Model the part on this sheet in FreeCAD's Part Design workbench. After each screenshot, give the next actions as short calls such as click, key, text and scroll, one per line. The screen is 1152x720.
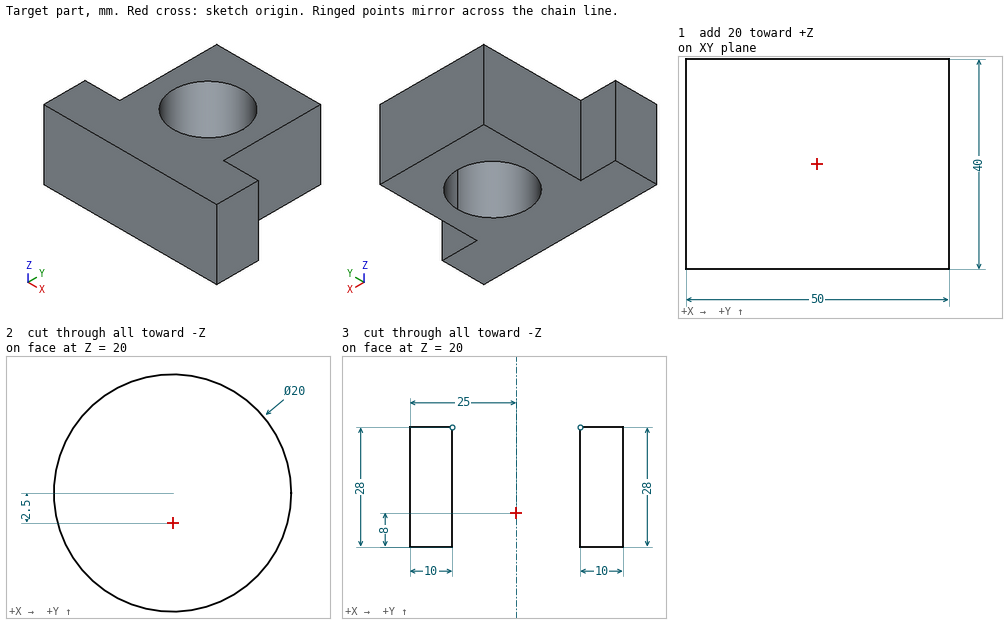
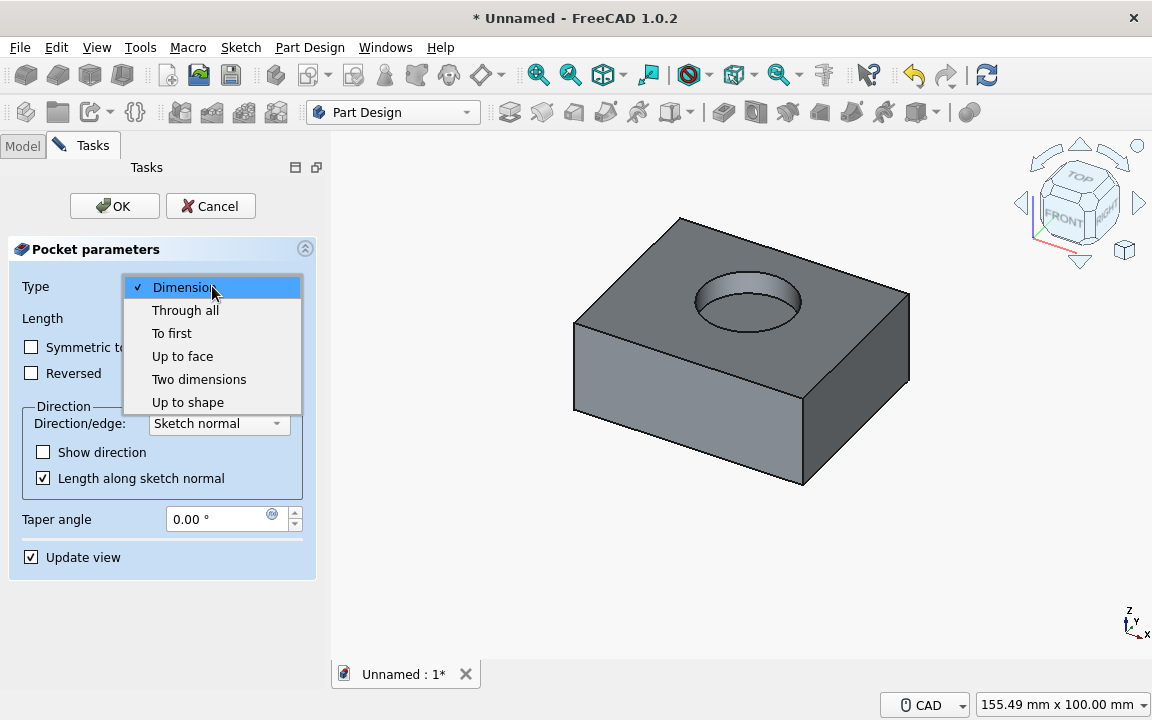
click(212, 310)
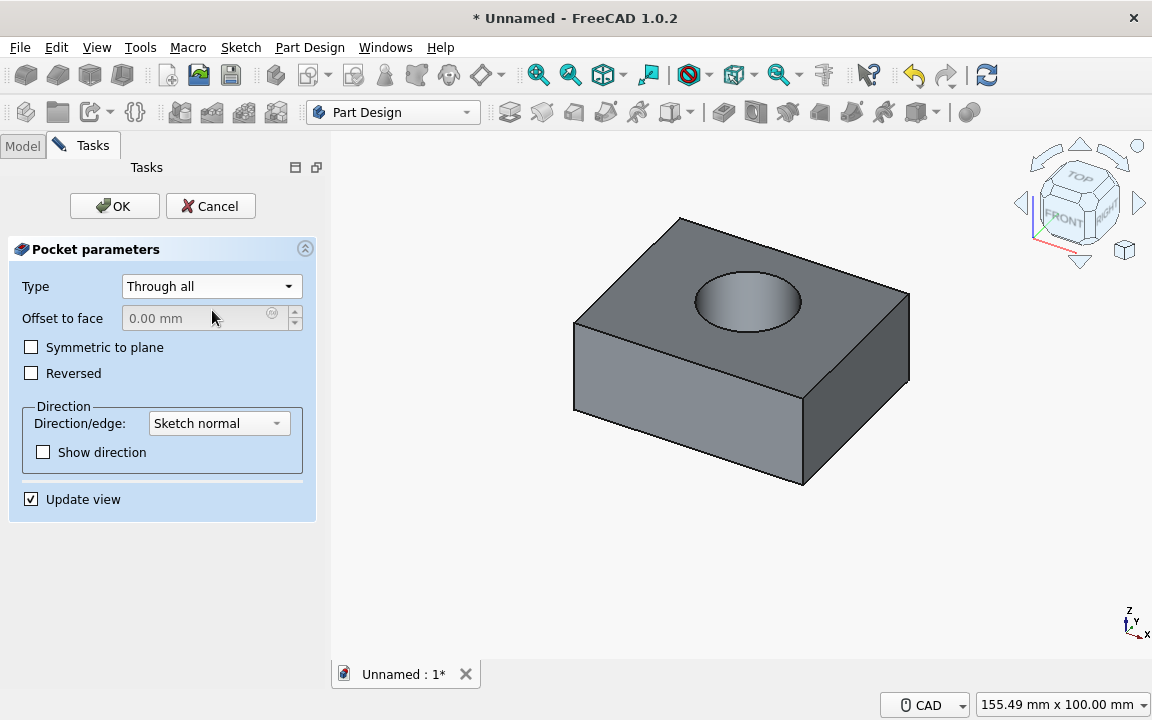
click(115, 206)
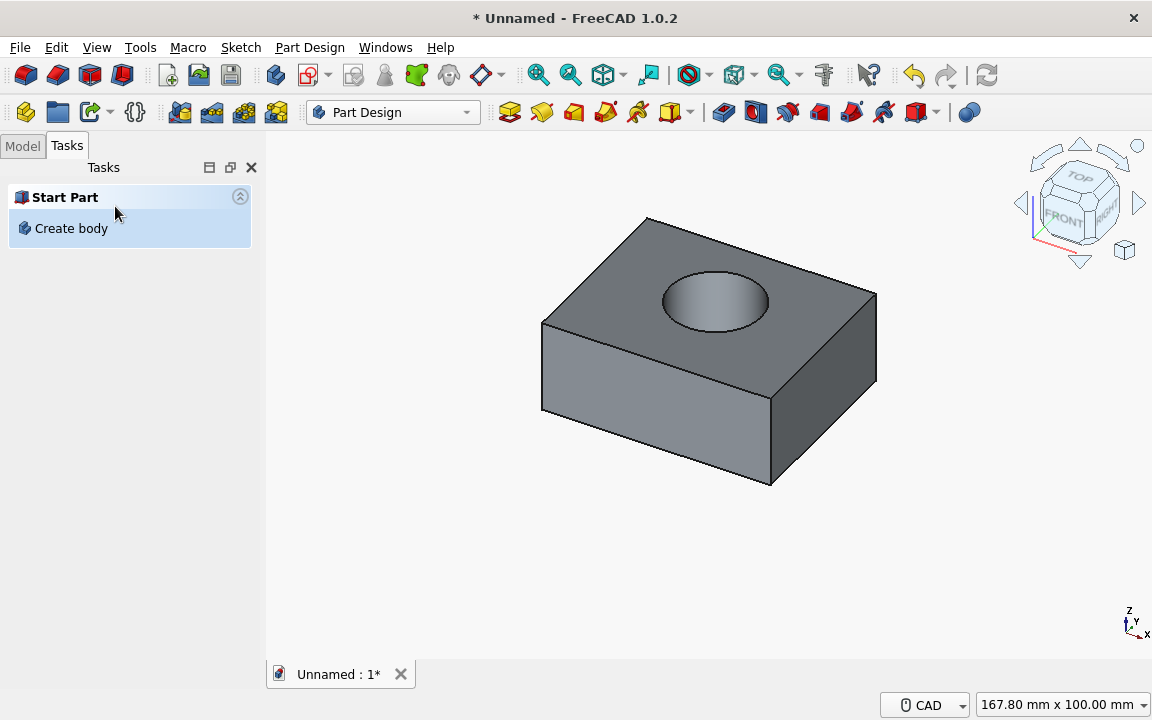
click(744, 359)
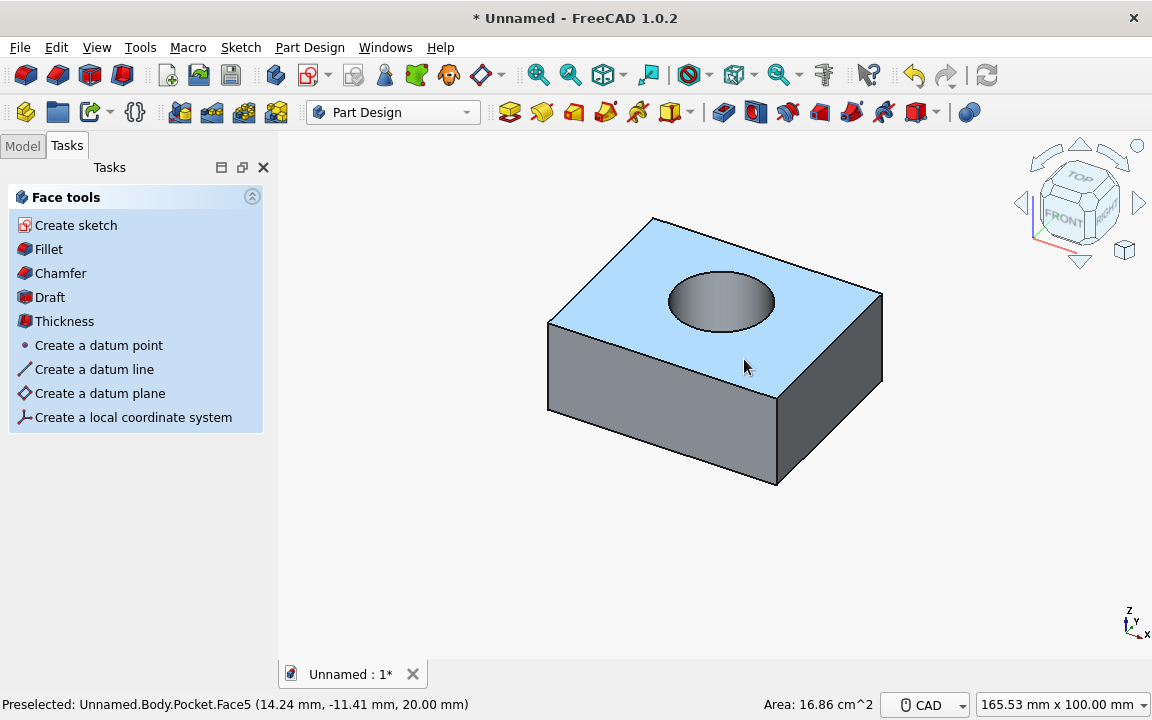
click(308, 76)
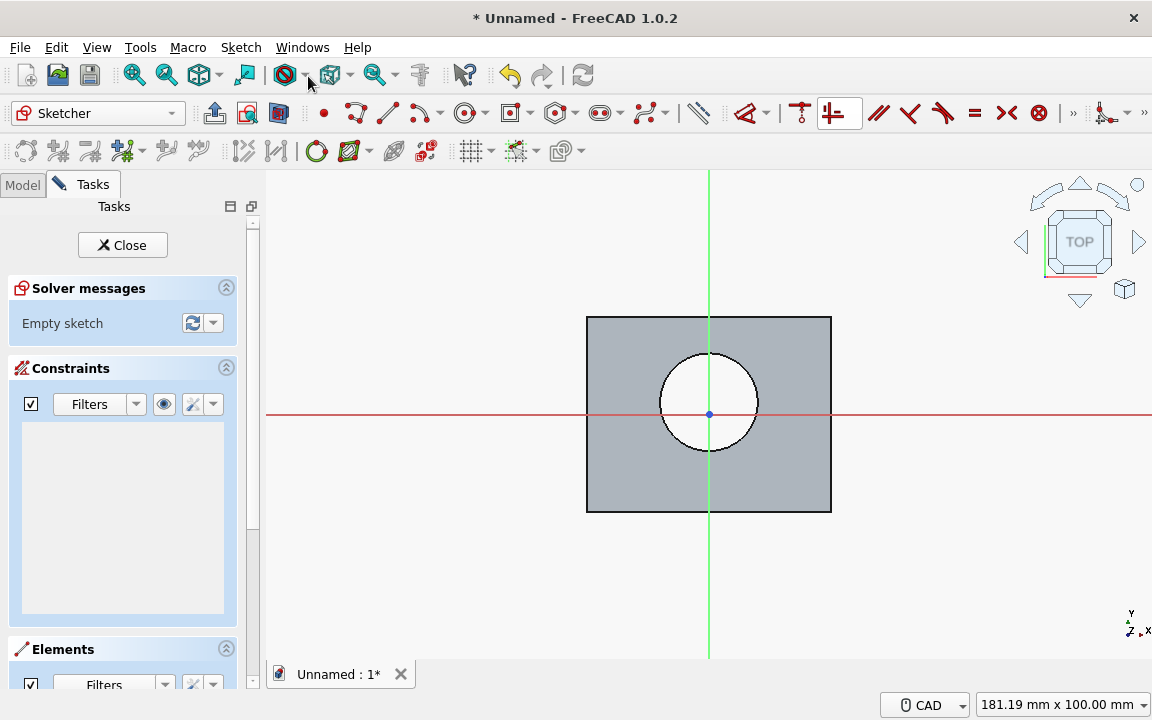
scroll(792, 349, up, 3)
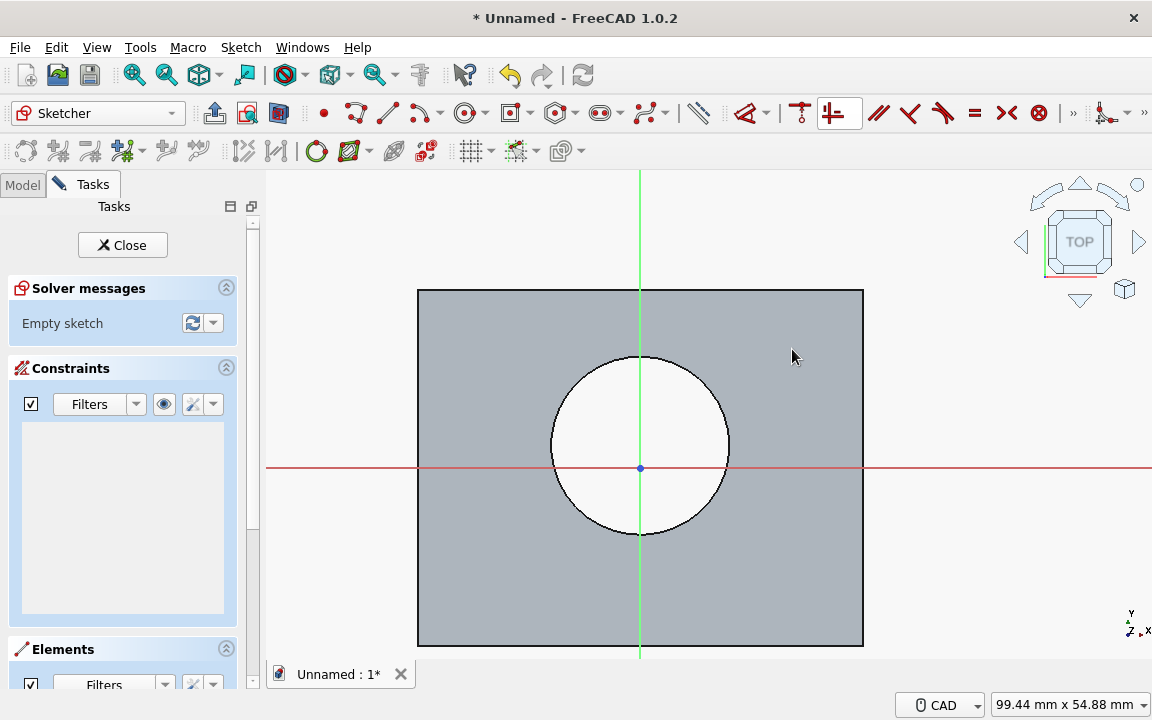
click(532, 114)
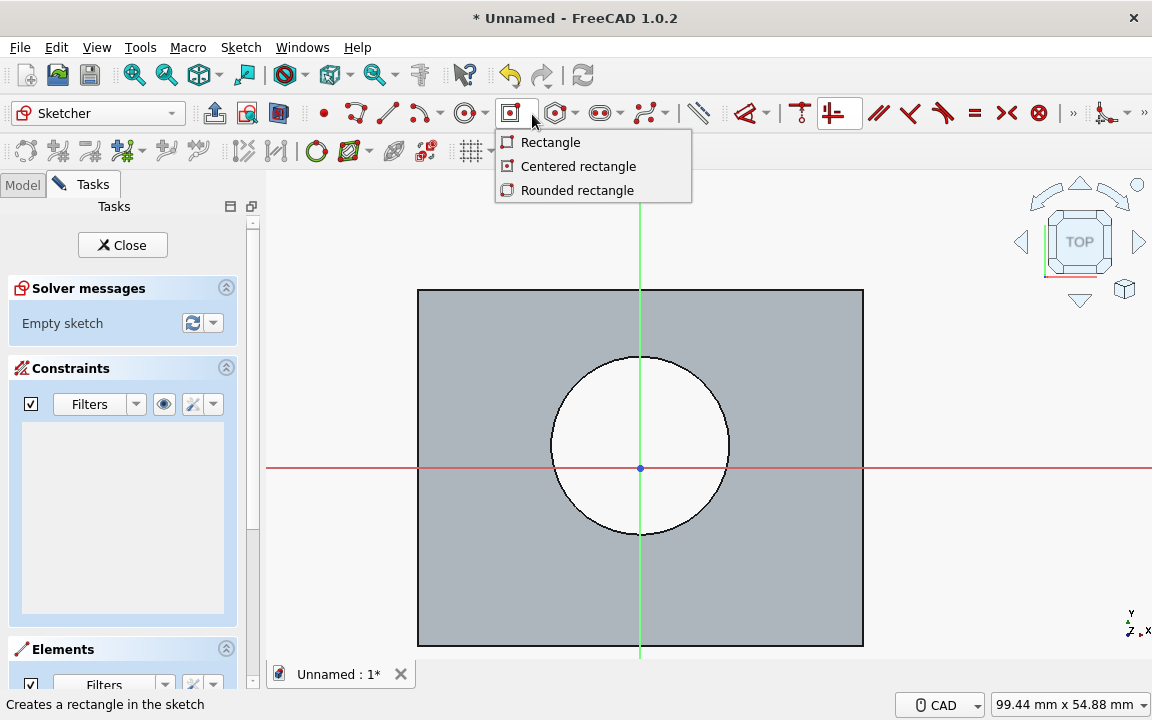
click(594, 142)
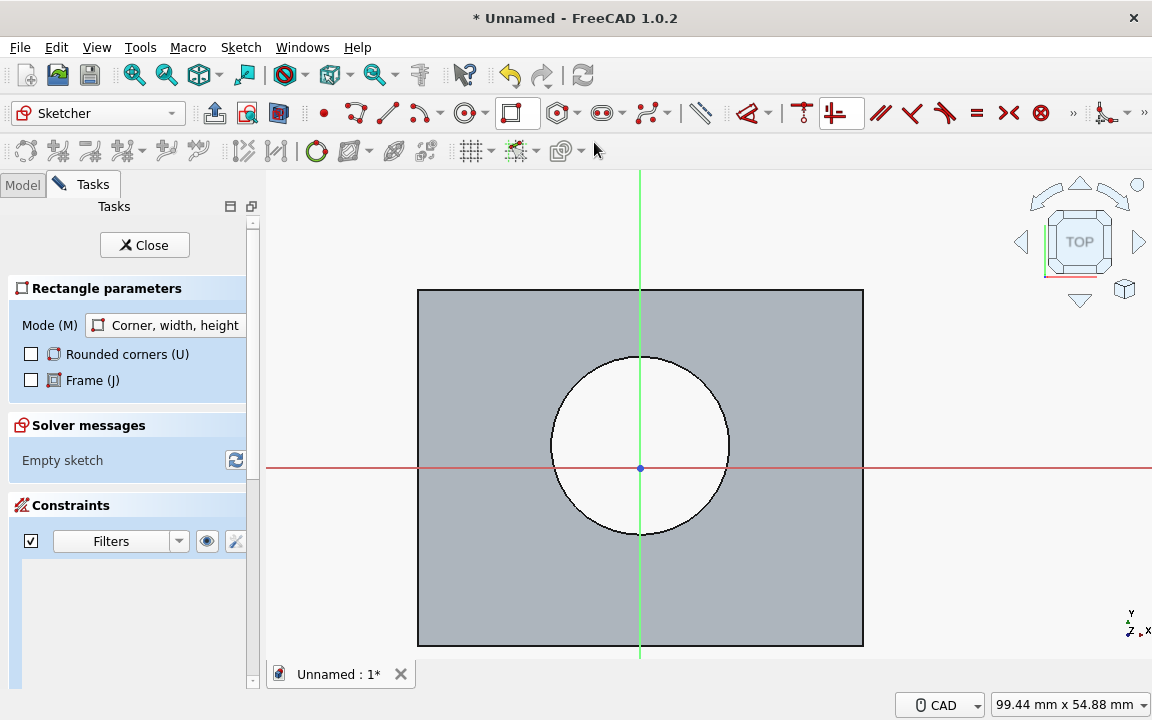
click(418, 290)
move(507, 539)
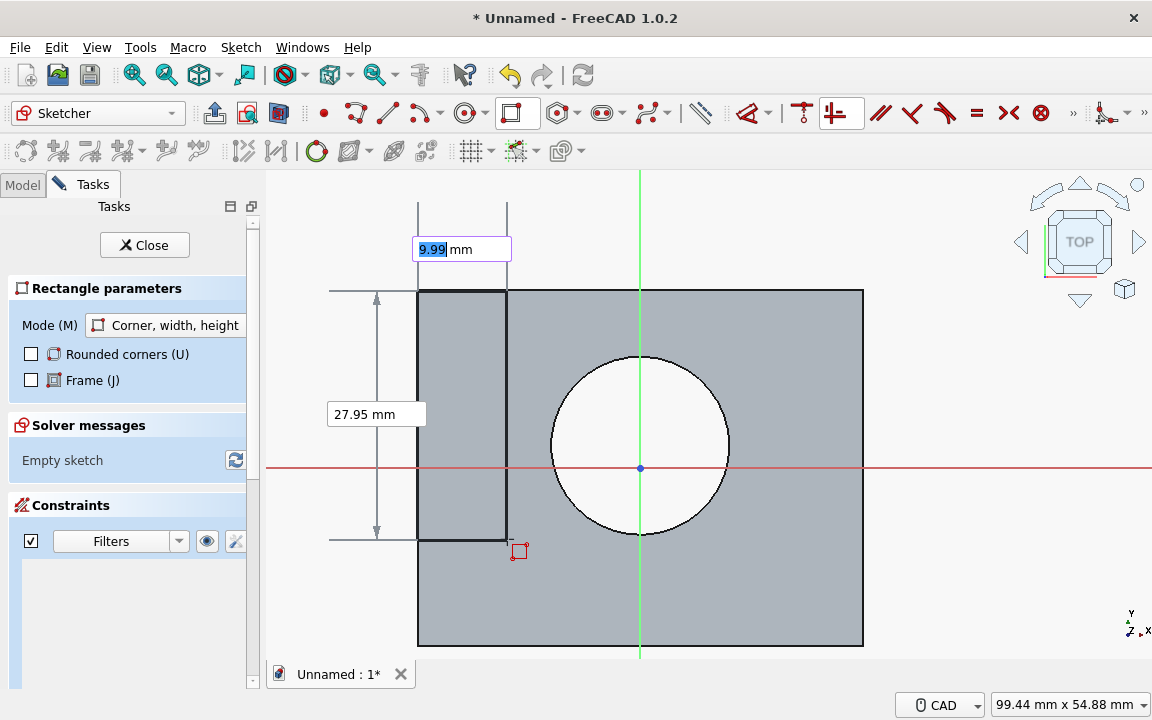
text(10)
key(Tab)
text(28)
key(Return)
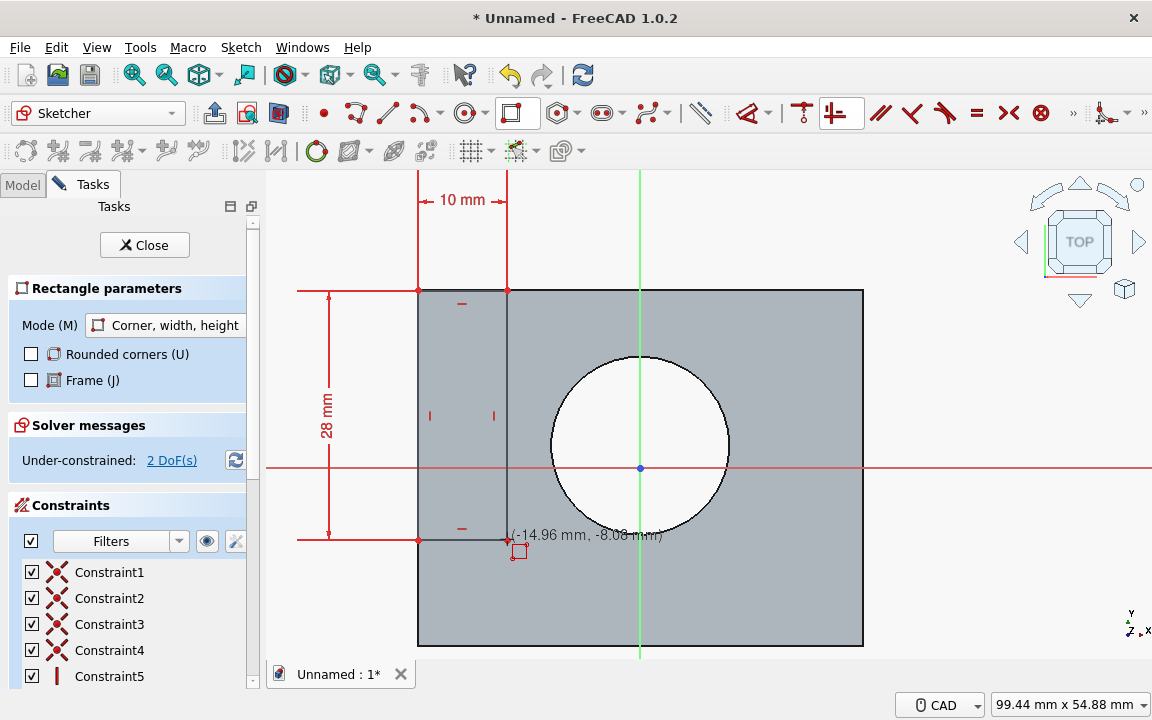
click(774, 290)
move(863, 539)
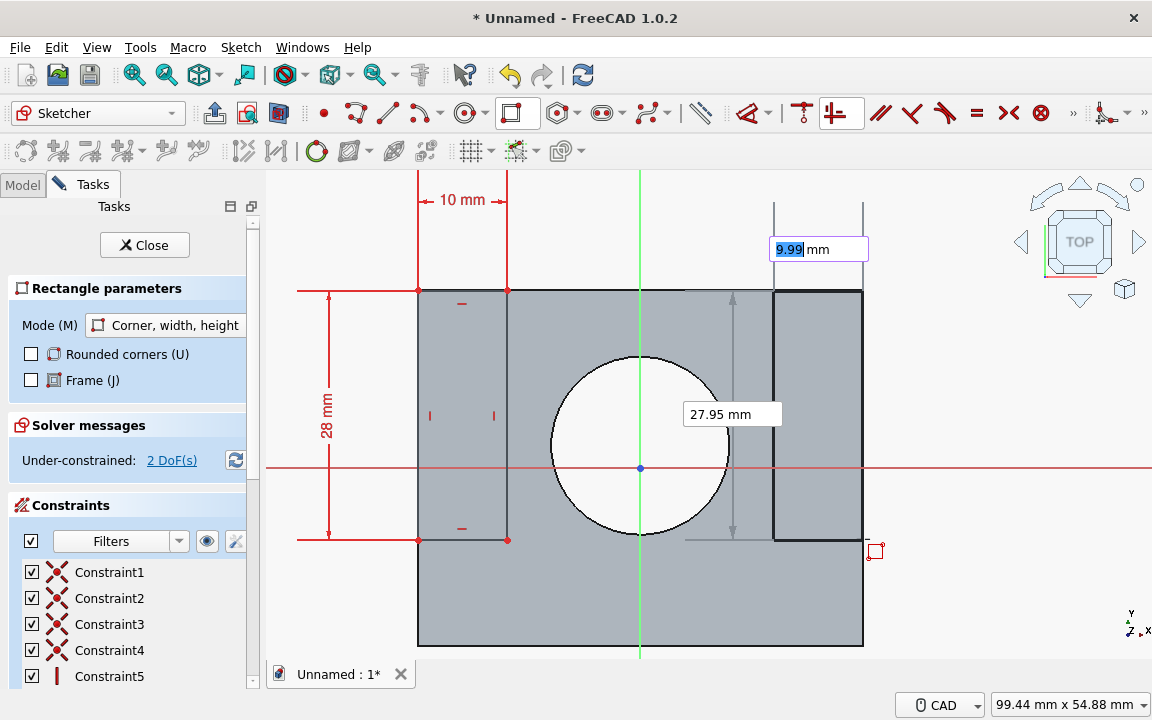
text(10)
key(Tab)
text(28)
key(Return)
key(Escape)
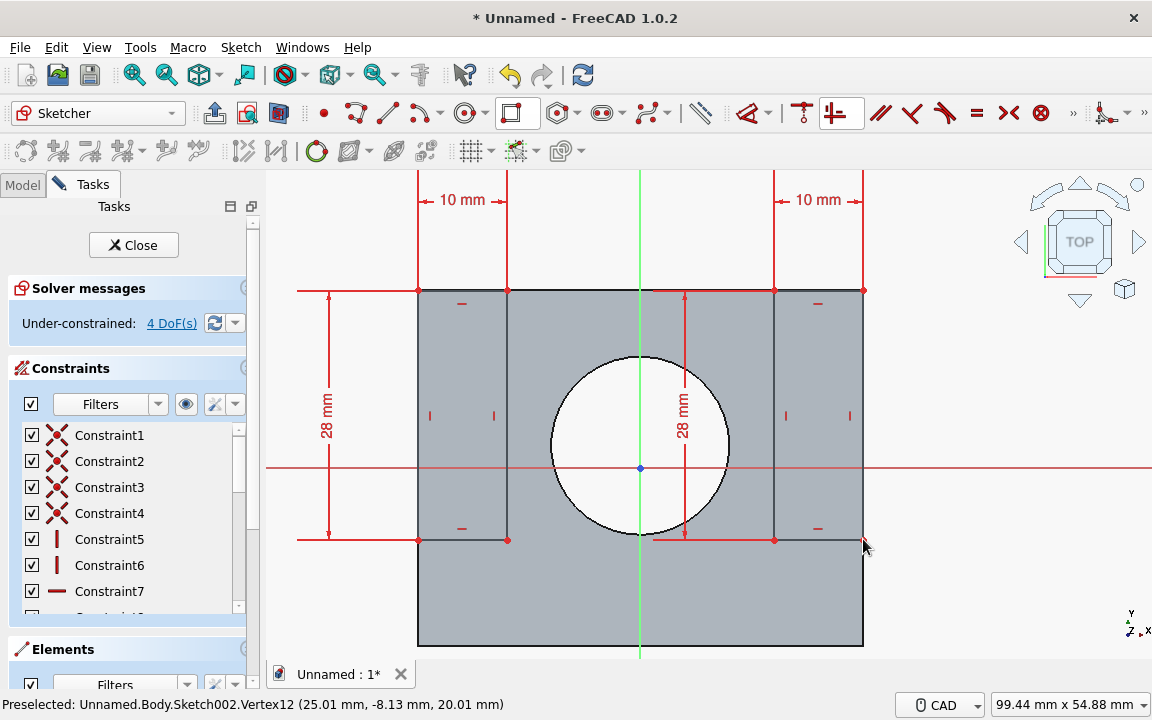
click(507, 291)